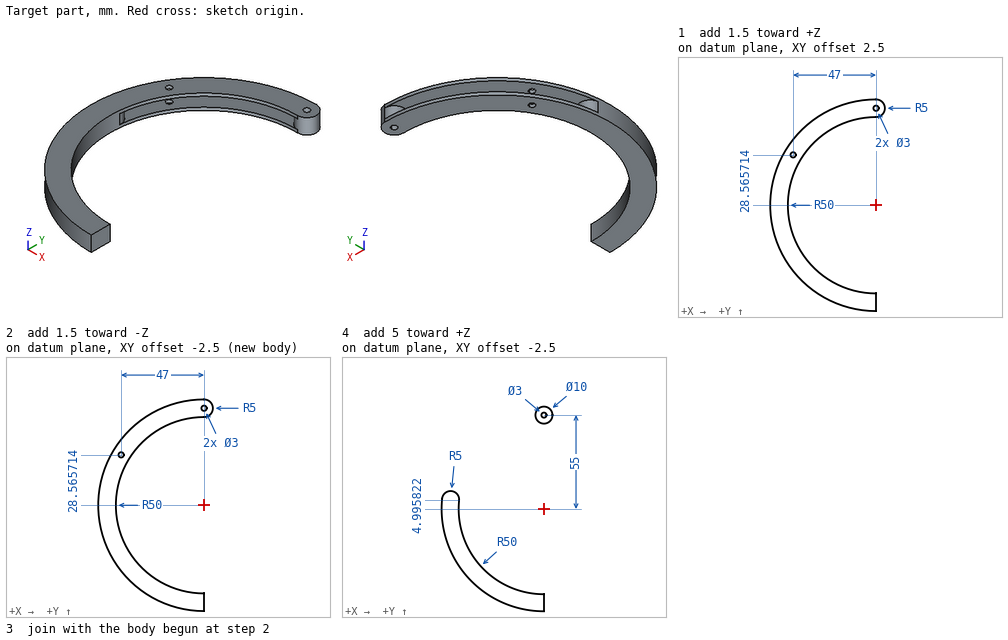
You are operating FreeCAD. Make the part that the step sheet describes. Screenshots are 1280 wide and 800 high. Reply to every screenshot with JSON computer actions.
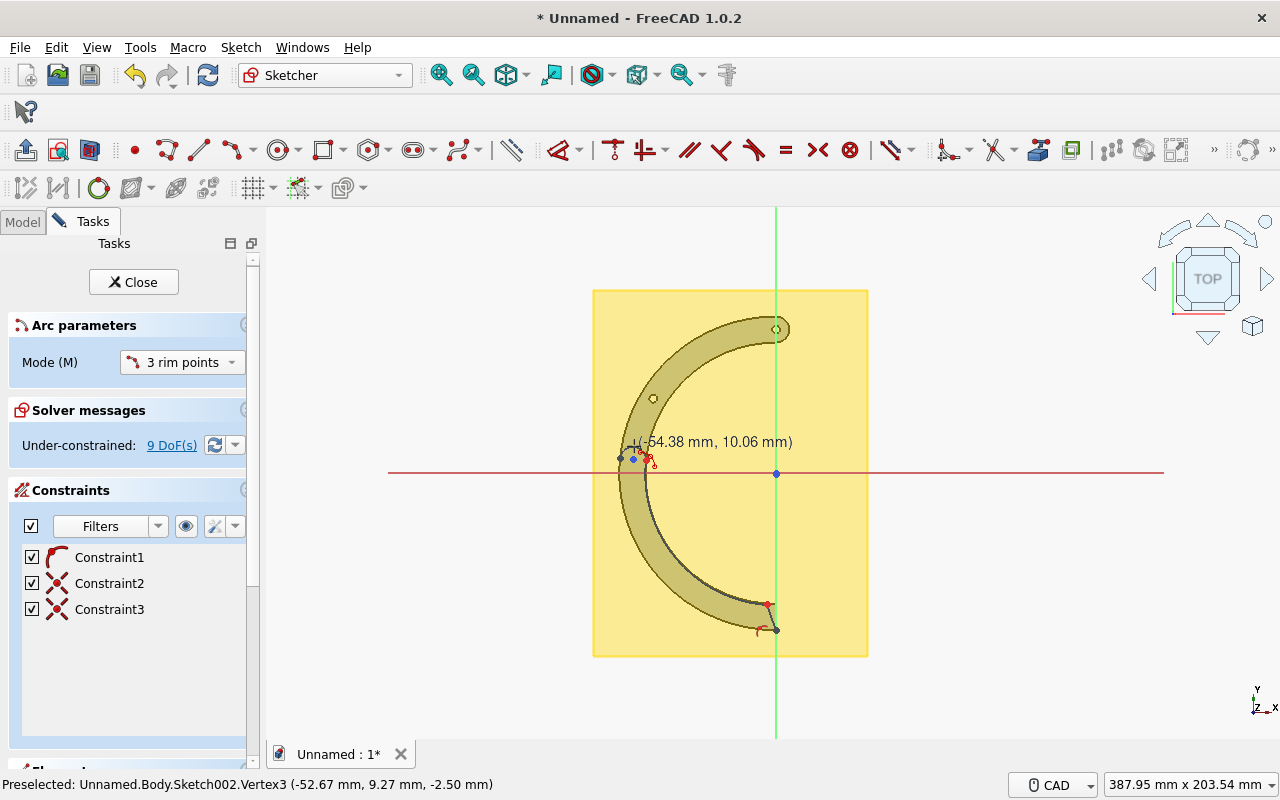
{"action": "left_click", "coordinate": [620, 459]}
{"action": "left_click", "coordinate": [776, 631]}
{"action": "left_click", "coordinate": [660, 579]}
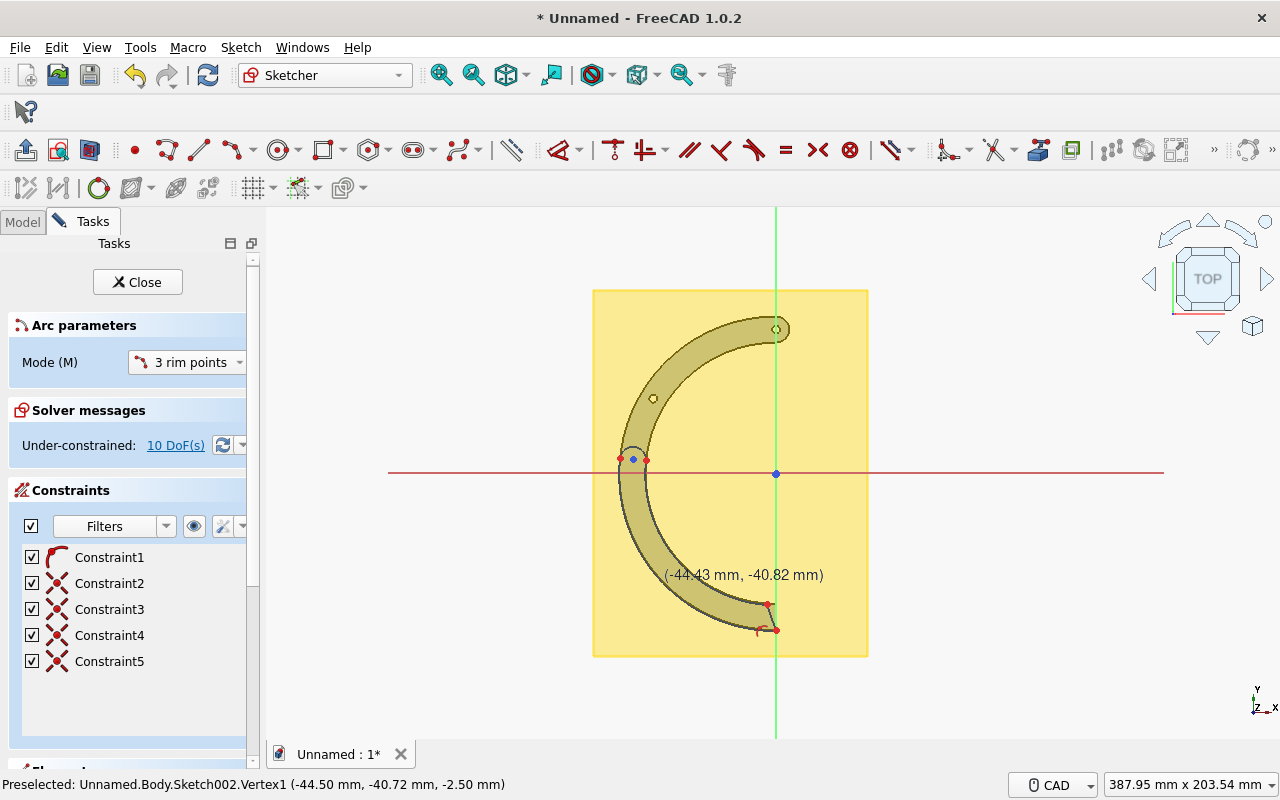
{"action": "left_click", "coordinate": [278, 150]}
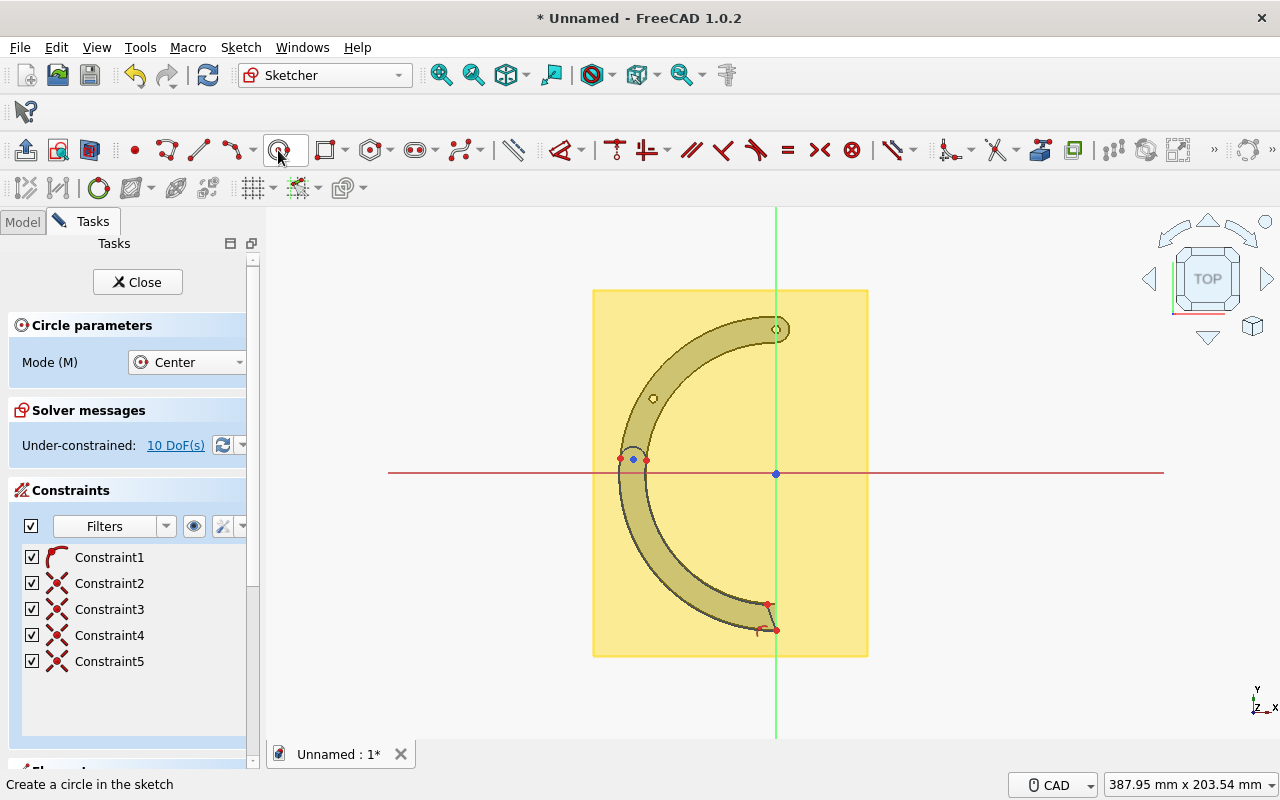
{"action": "scroll", "coordinate": [776, 330], "scroll_direction": "up", "scroll_amount": 3}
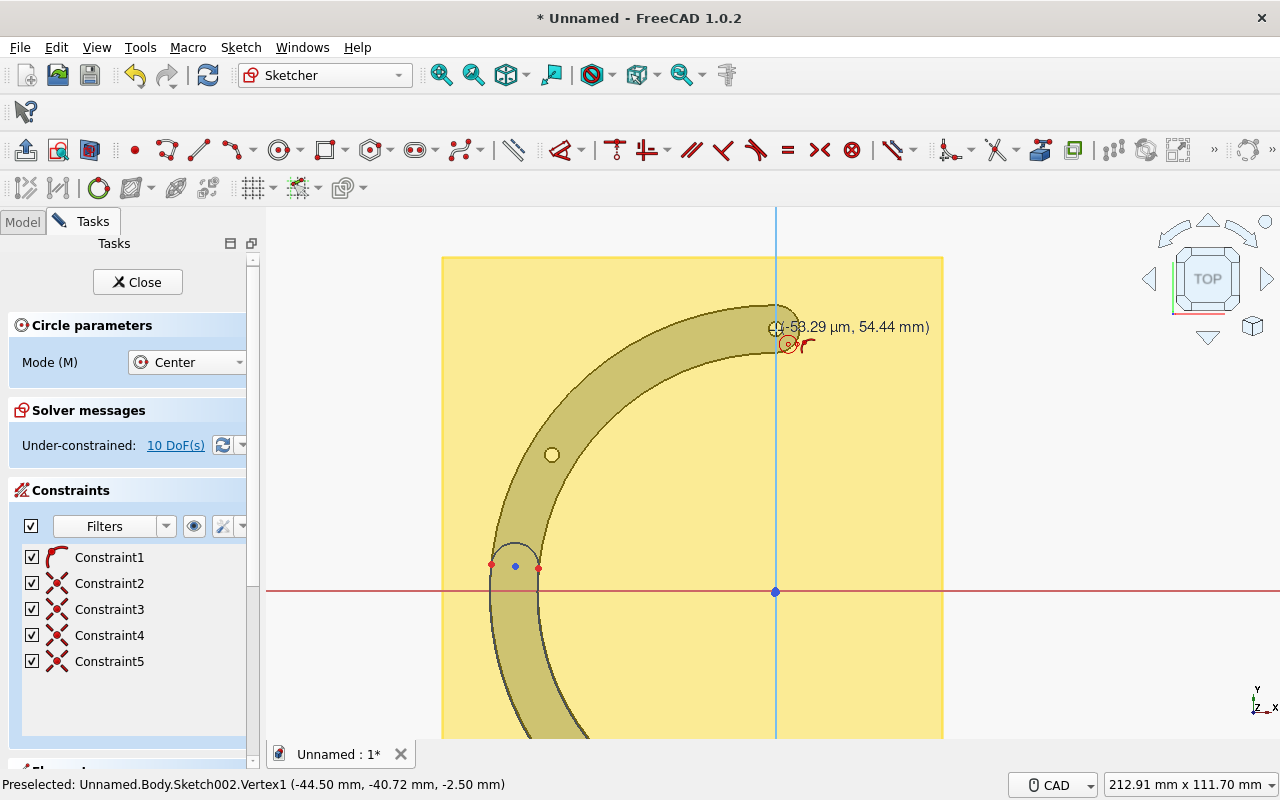
{"action": "left_click", "coordinate": [776, 329]}
{"action": "left_click", "coordinate": [793, 312]}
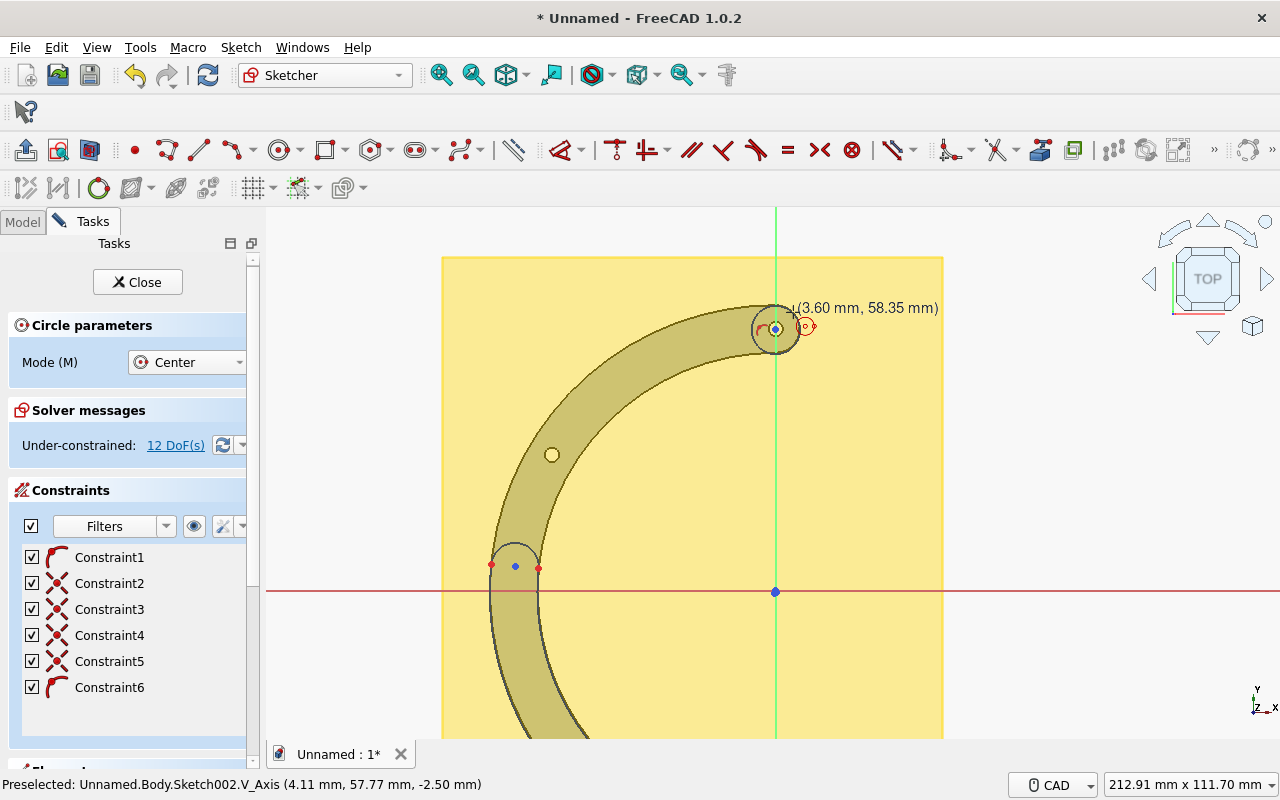
{"action": "scroll", "coordinate": [776, 329], "scroll_direction": "up", "scroll_amount": 6}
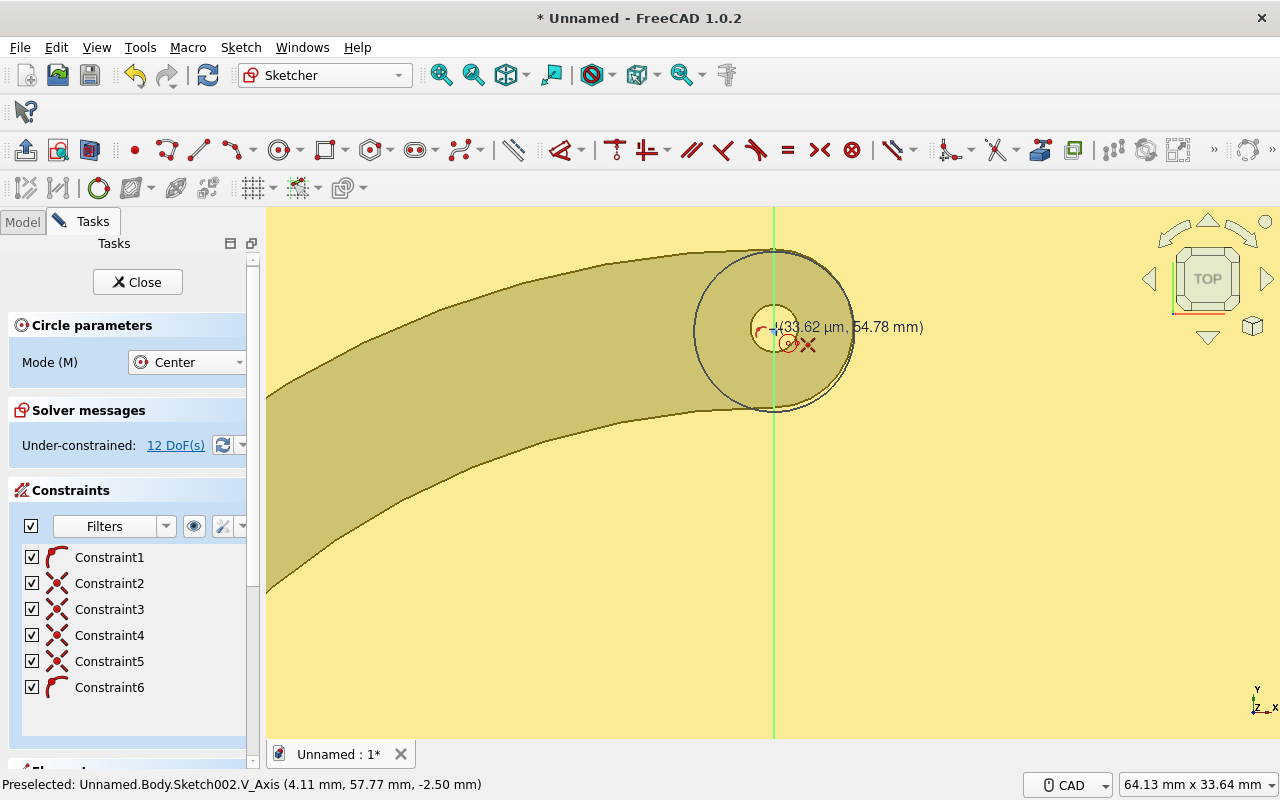
{"action": "scroll", "coordinate": [776, 329], "scroll_direction": "down", "scroll_amount": 9}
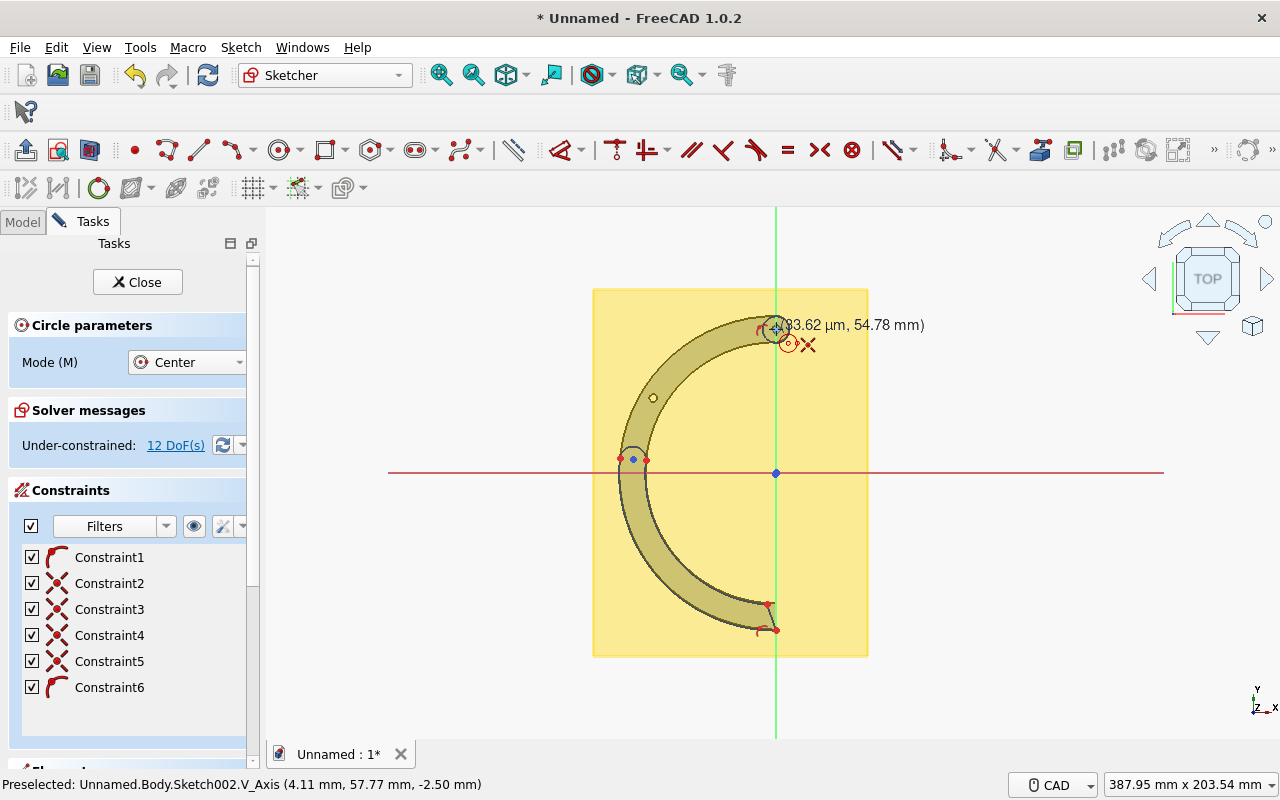
{"action": "left_click", "coordinate": [776, 330]}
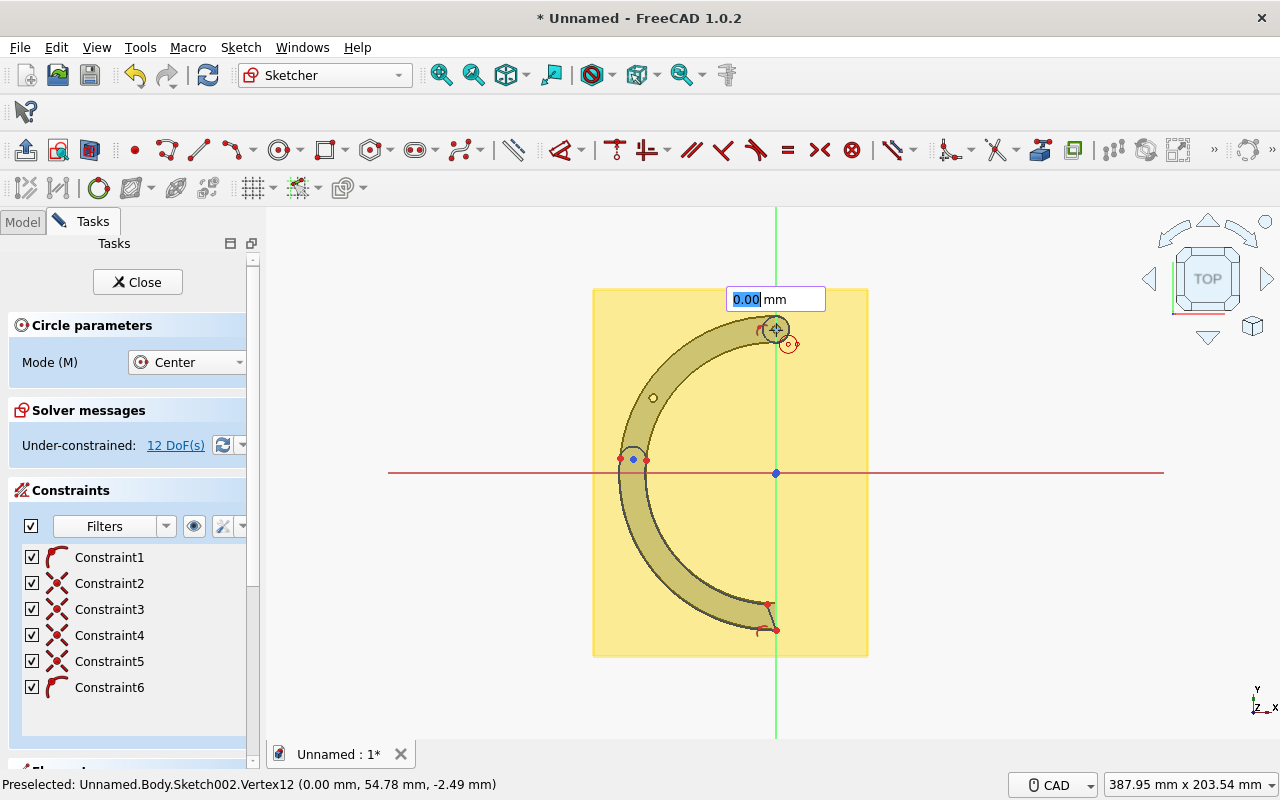
{"action": "scroll", "coordinate": [780, 328], "scroll_direction": "up", "scroll_amount": 8}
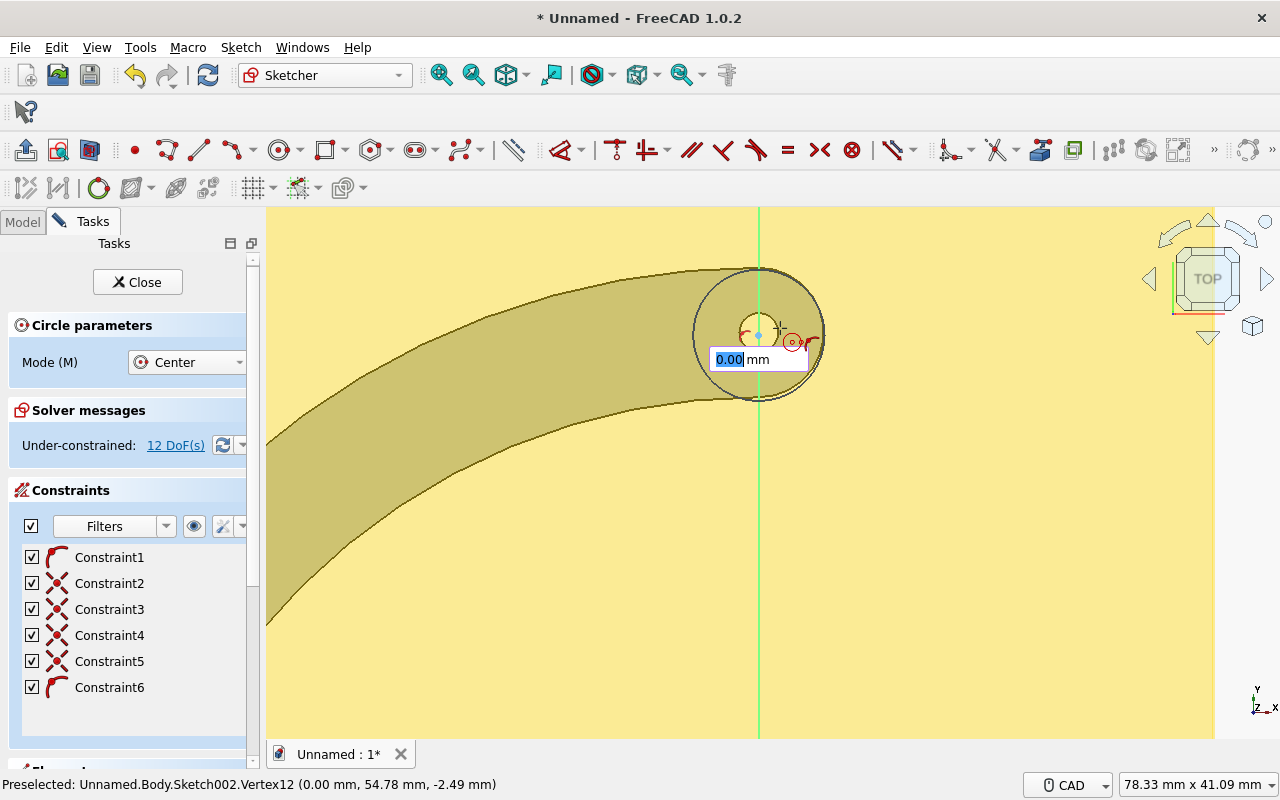
{"action": "left_click", "coordinate": [777, 326]}
{"action": "key", "text": "Escape"}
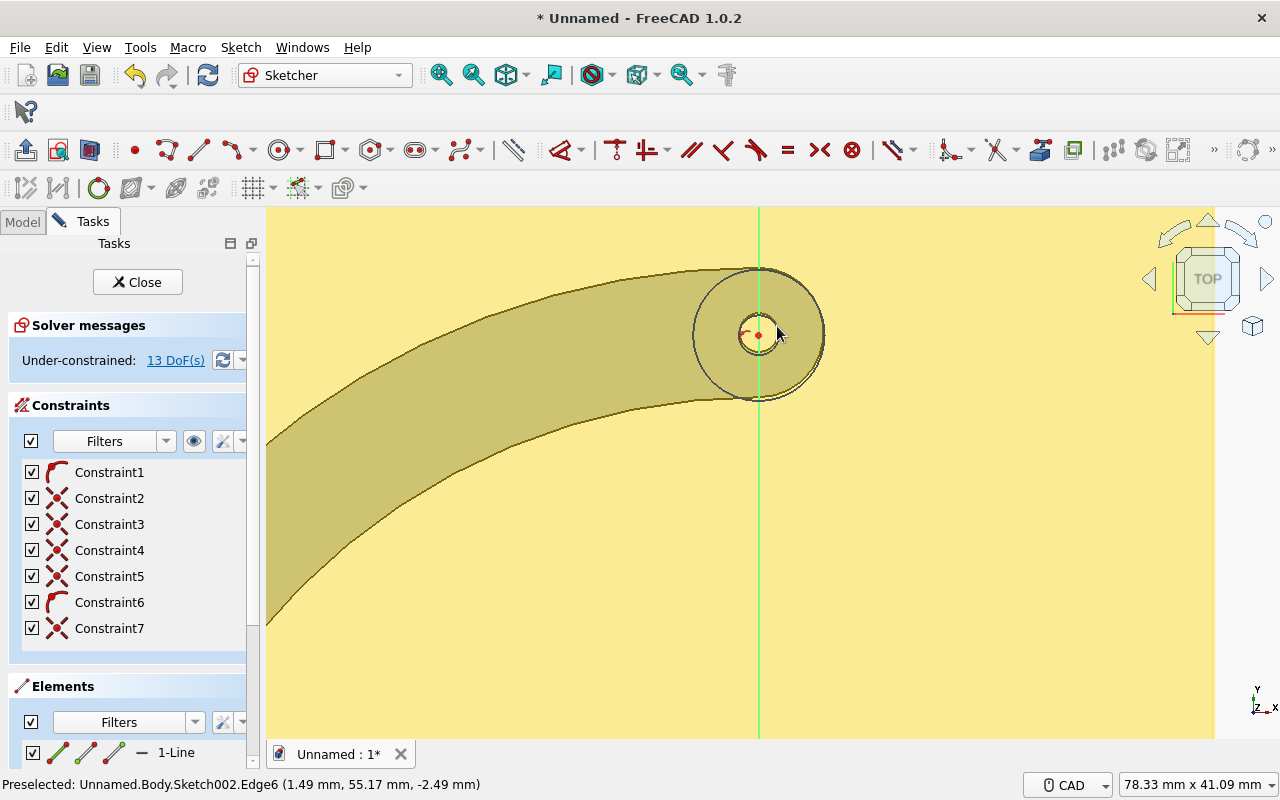
{"action": "scroll", "coordinate": [780, 328], "scroll_direction": "down", "scroll_amount": 8}